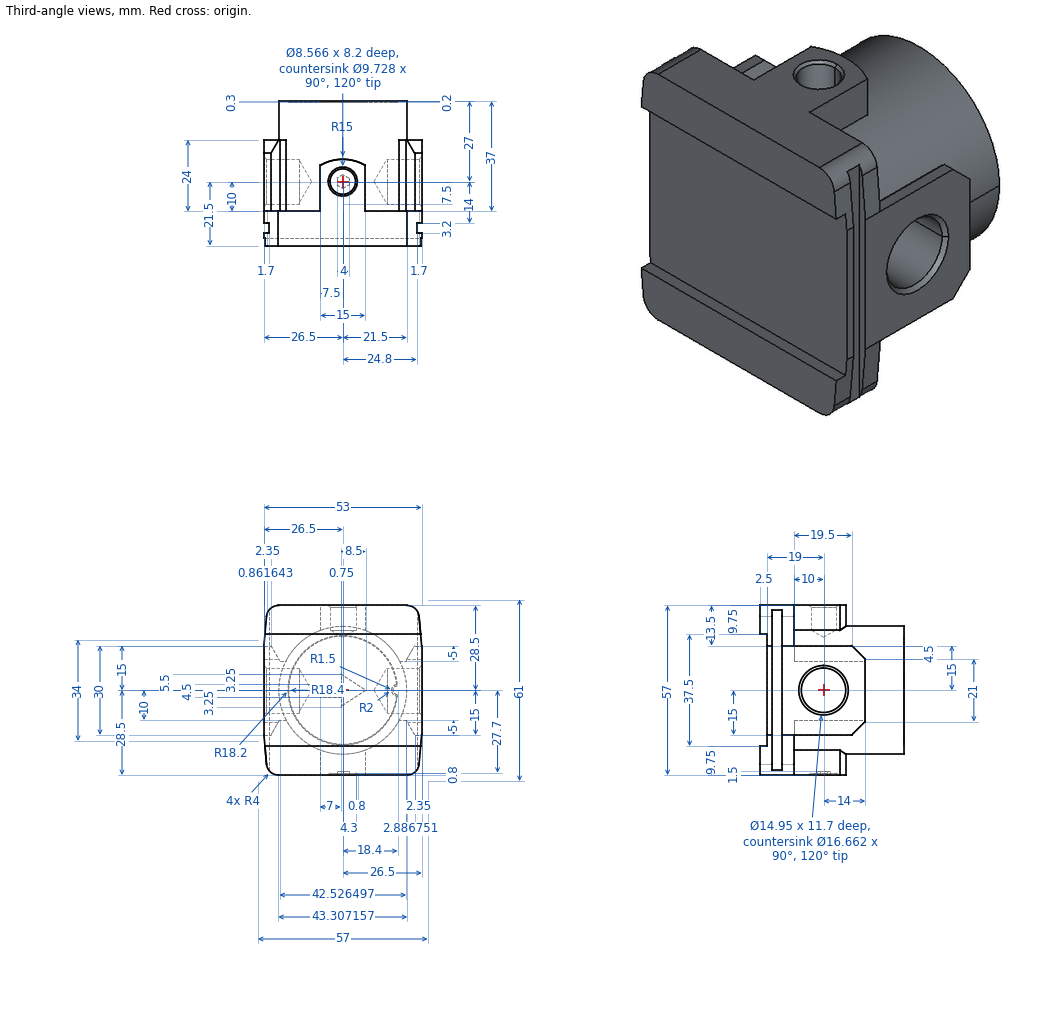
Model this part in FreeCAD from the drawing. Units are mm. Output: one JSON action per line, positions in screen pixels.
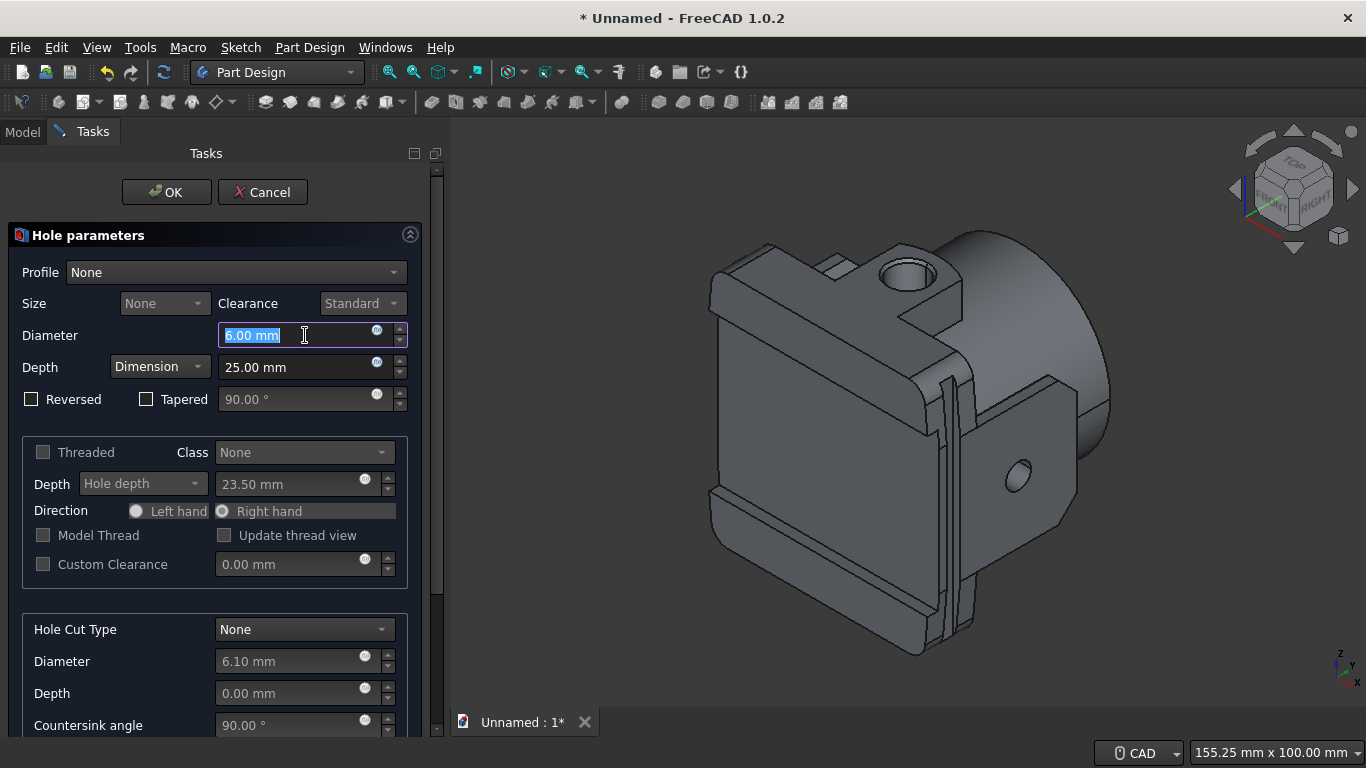
{"action": "type", "text": "14.95"}
{"action": "key", "text": "Tab"}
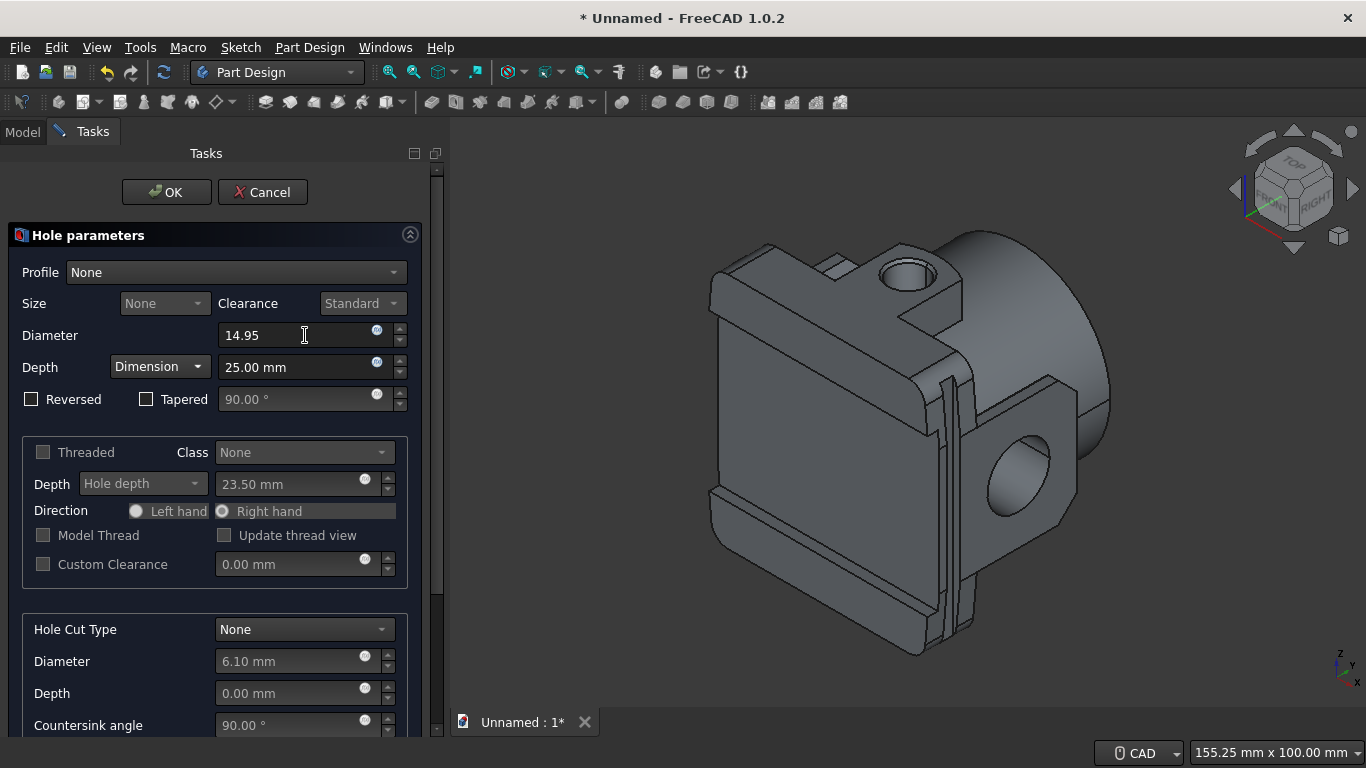
{"action": "triple_click", "coordinate": [305, 367]}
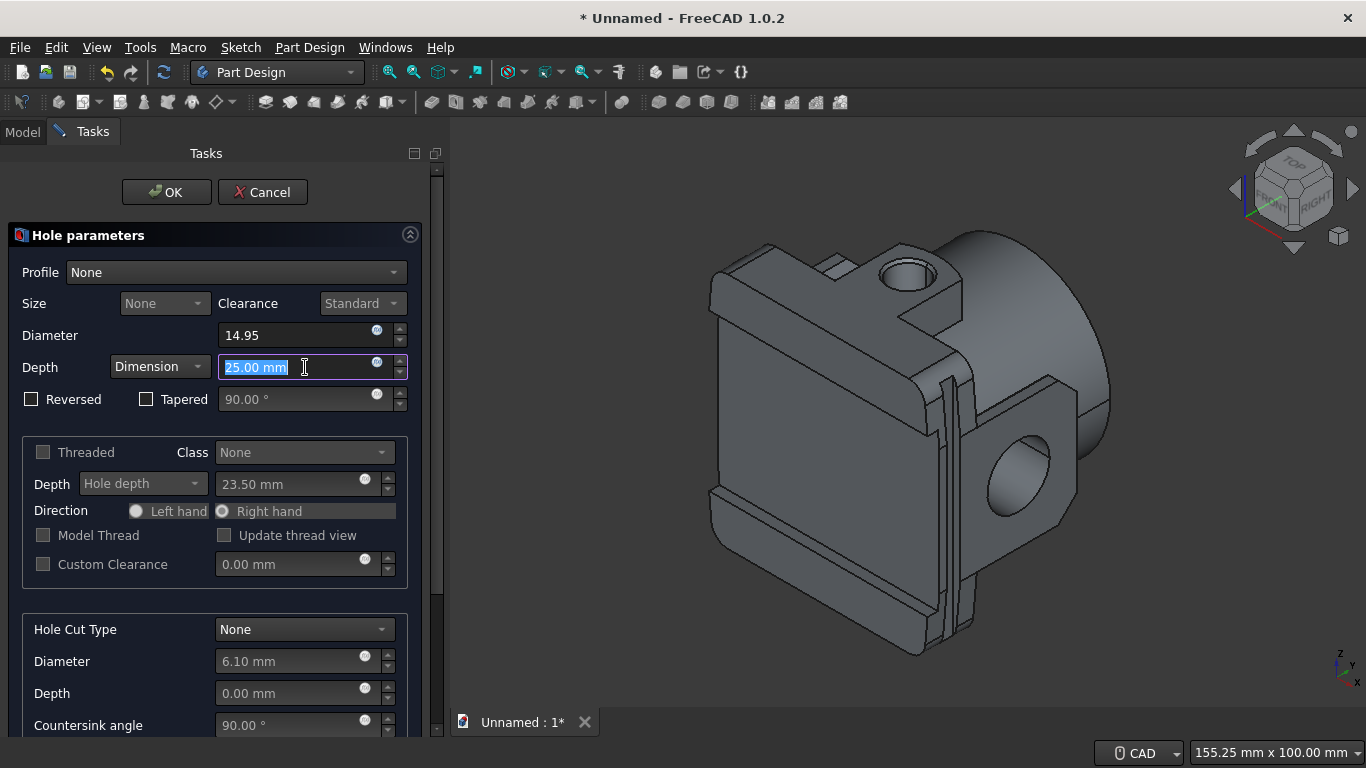
{"action": "type", "text": "11.7"}
{"action": "key", "text": "Tab"}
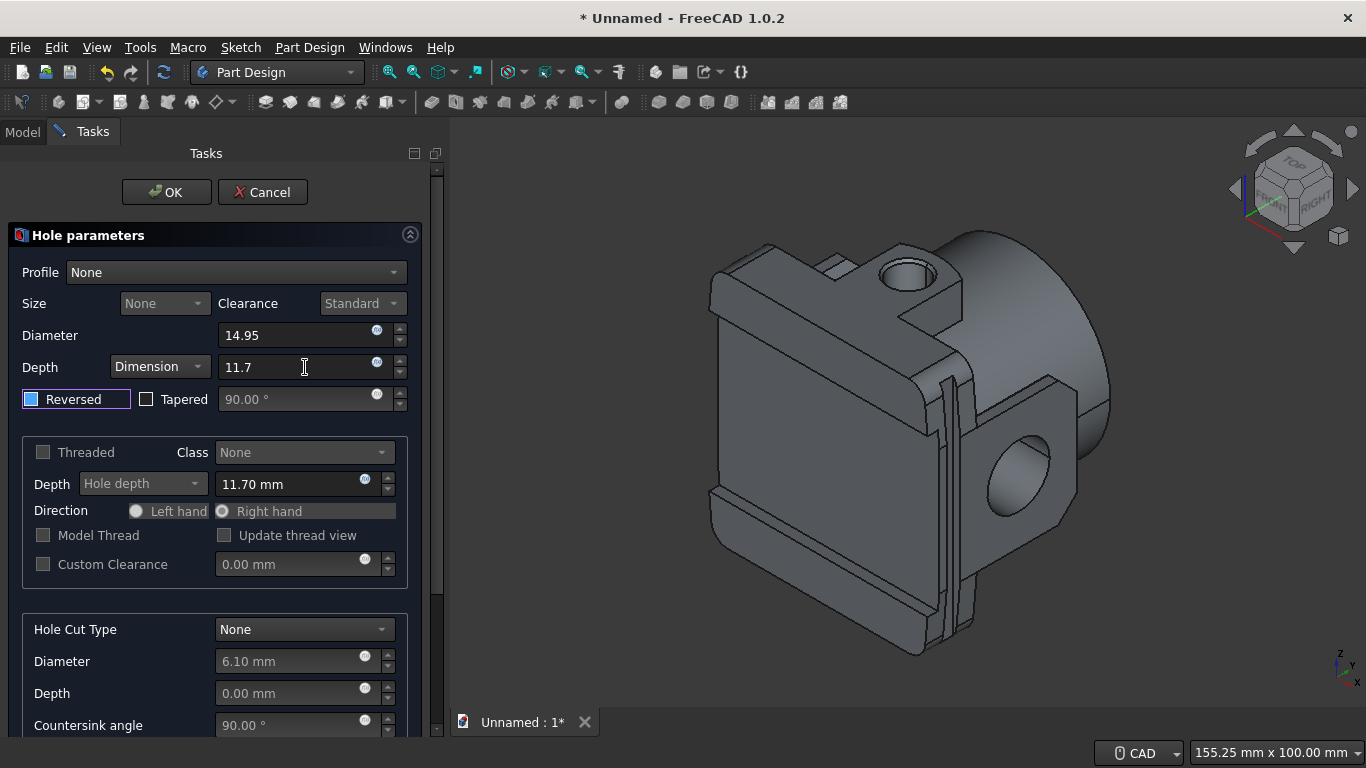
{"action": "left_click", "coordinate": [306, 630]}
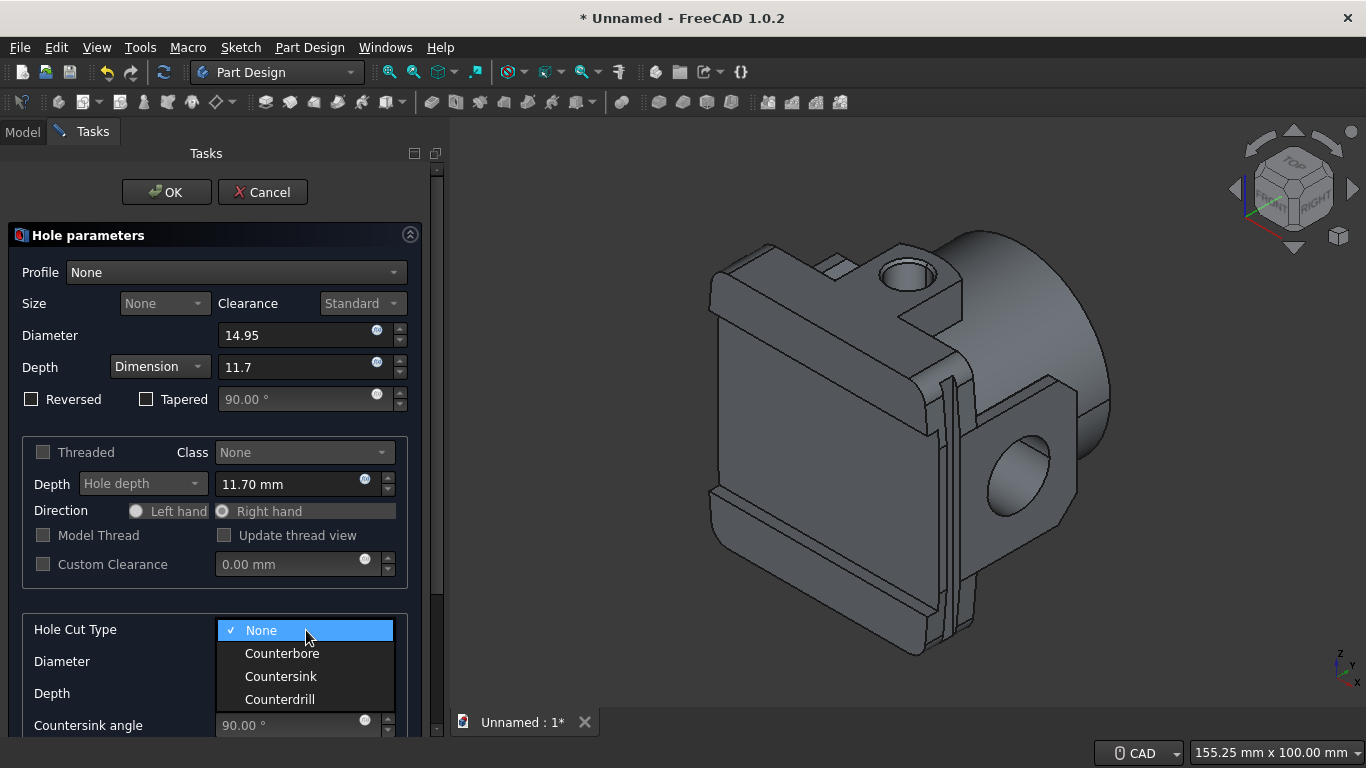
{"action": "left_click", "coordinate": [304, 676]}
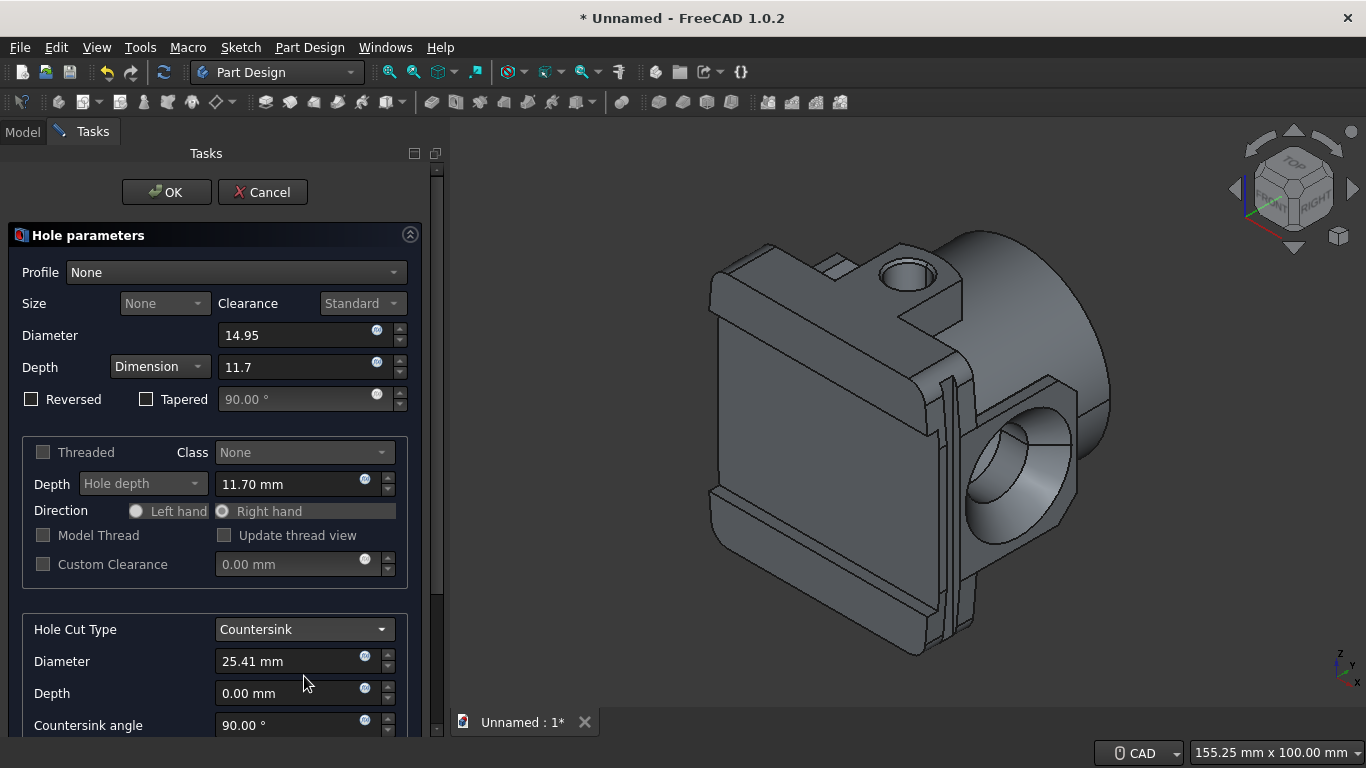
{"action": "triple_click", "coordinate": [298, 661]}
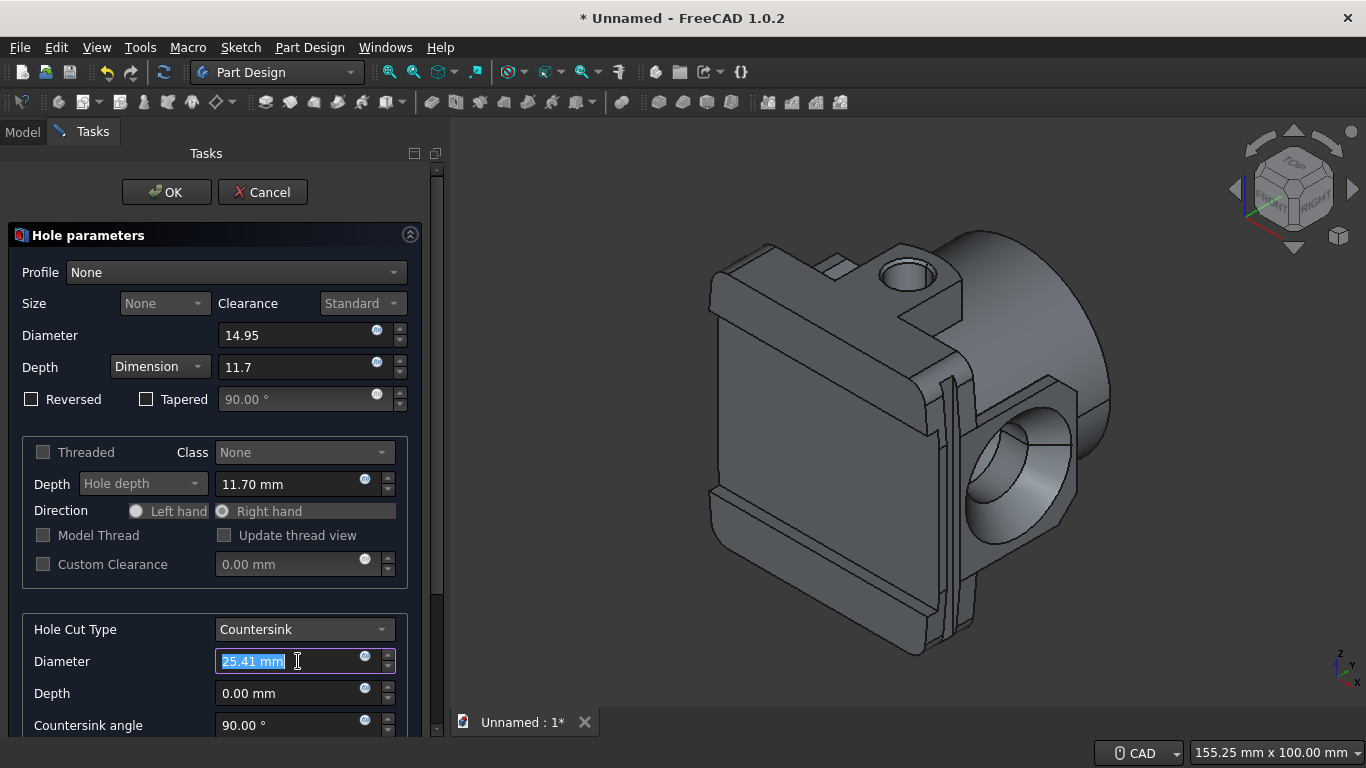
{"action": "type", "text": "16.662"}
{"action": "key", "text": "Tab"}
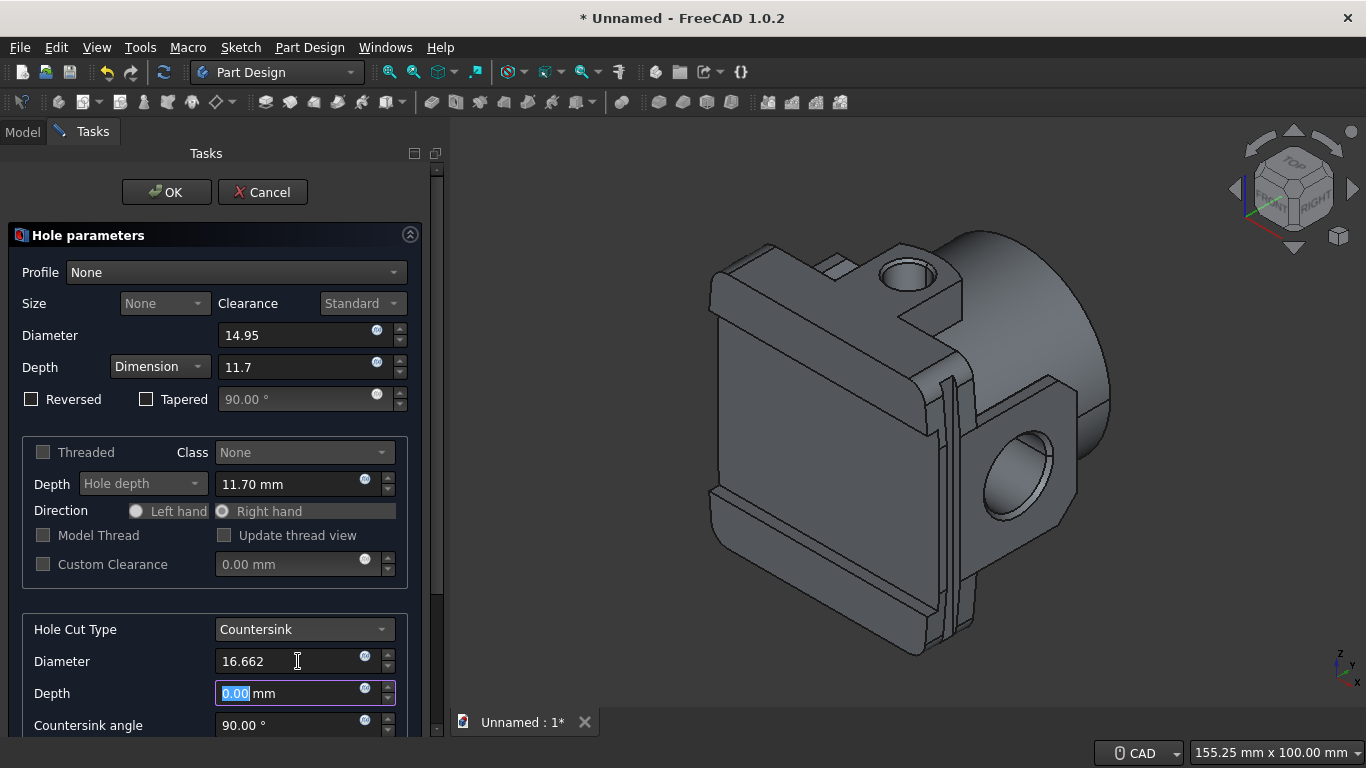
{"action": "scroll", "coordinate": [437, 450], "scroll_direction": "down", "scroll_amount": 3}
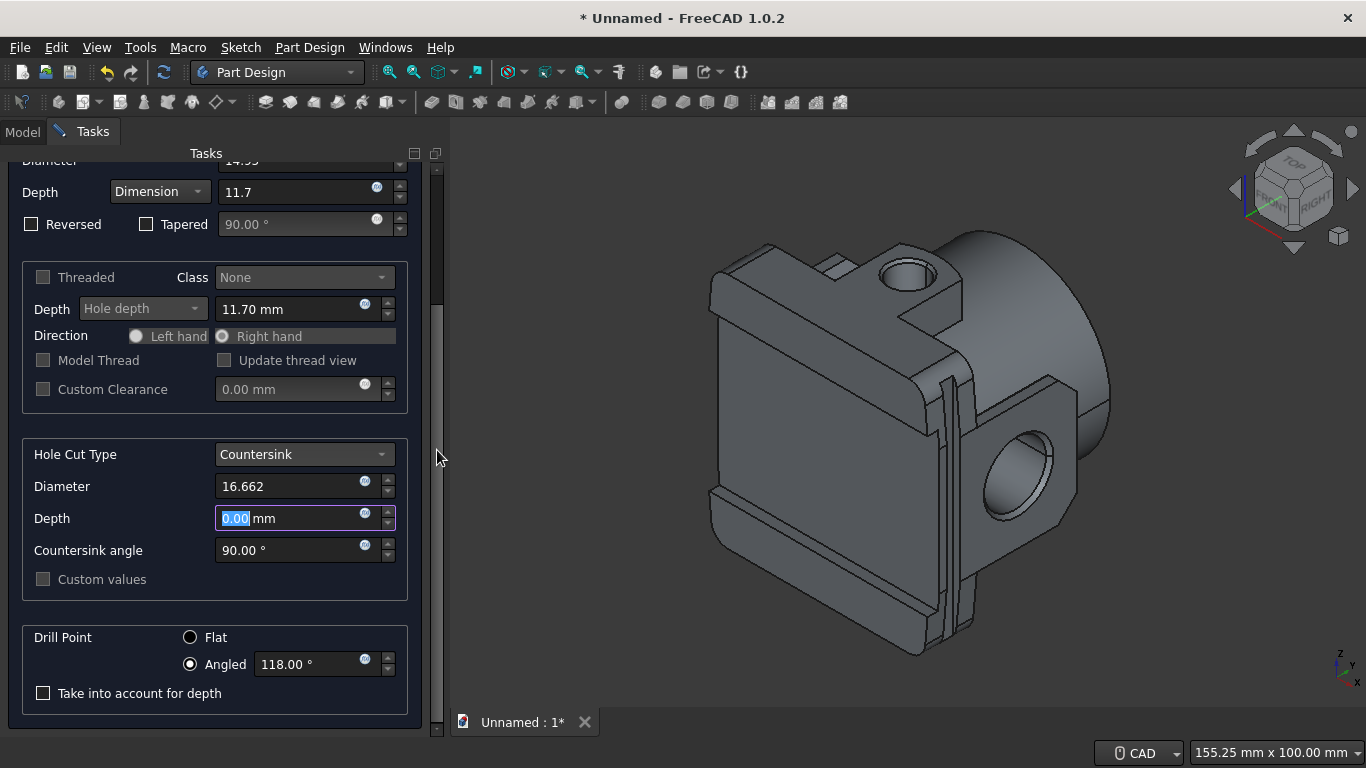
{"action": "triple_click", "coordinate": [317, 664]}